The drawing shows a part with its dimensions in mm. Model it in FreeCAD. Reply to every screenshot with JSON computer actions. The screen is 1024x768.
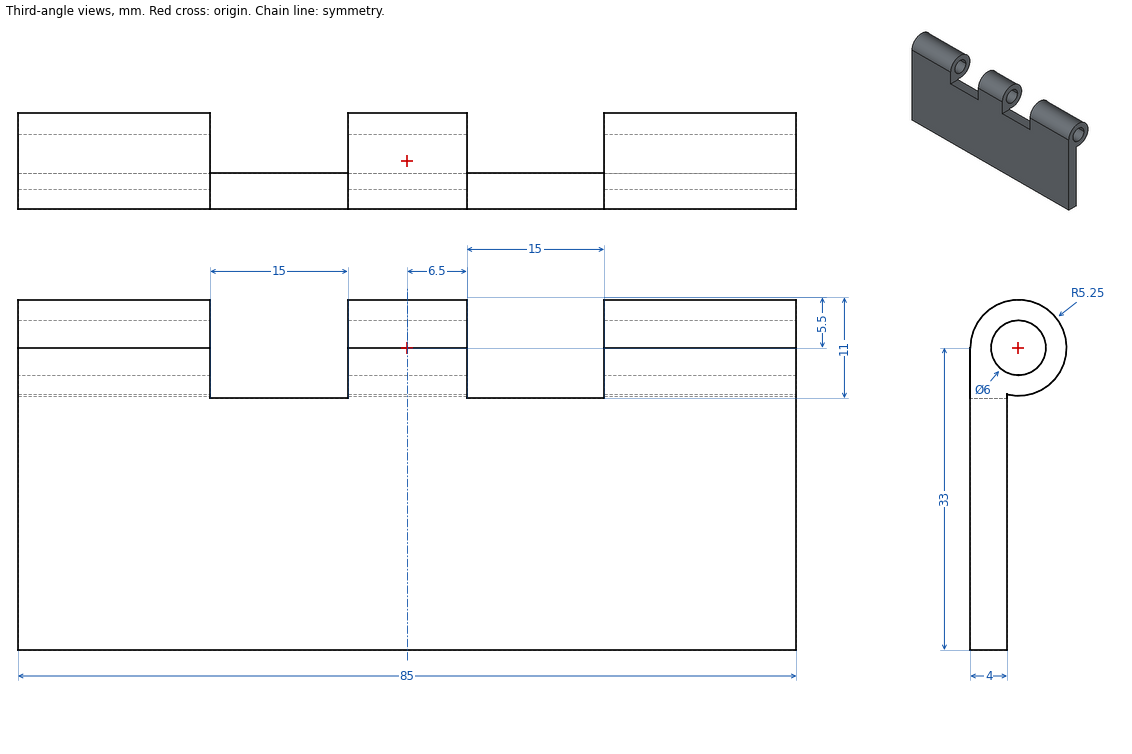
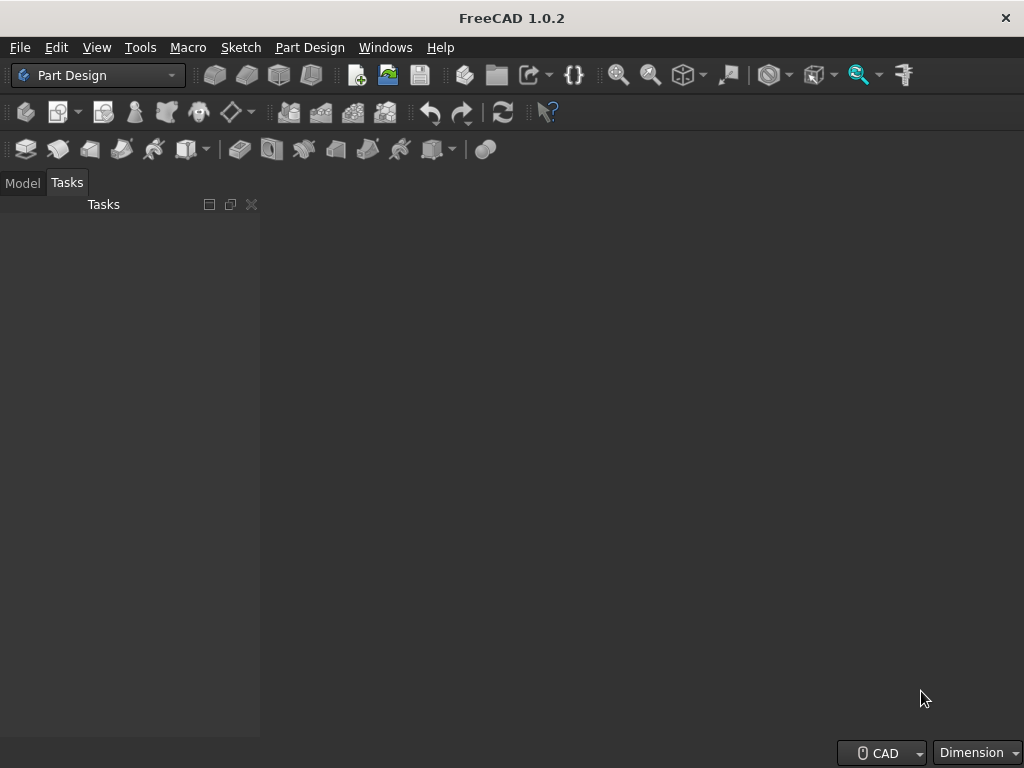
{"action": "left_click", "coordinate": [356, 76]}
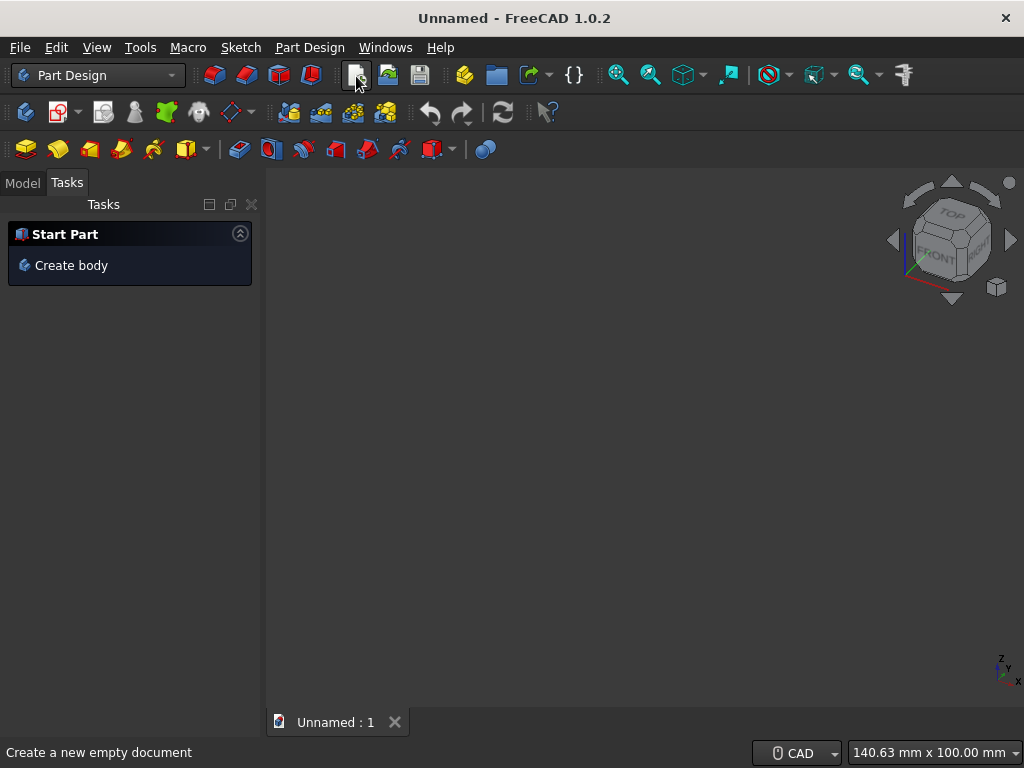
{"action": "left_click", "coordinate": [58, 112]}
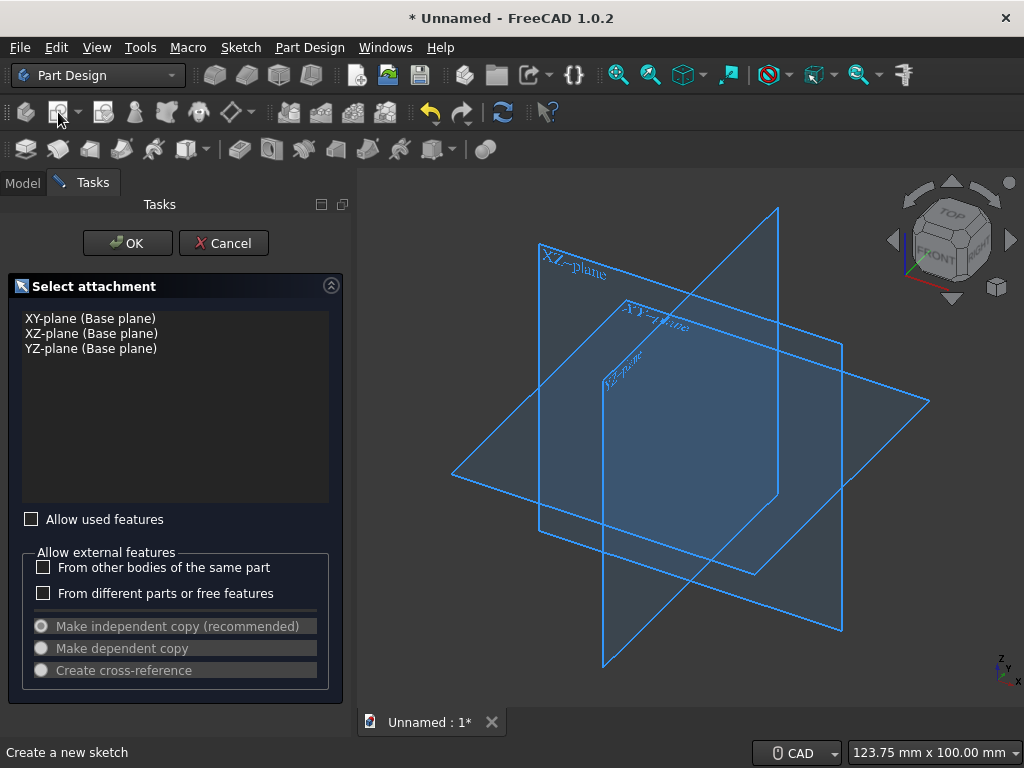
{"action": "left_click", "coordinate": [82, 348]}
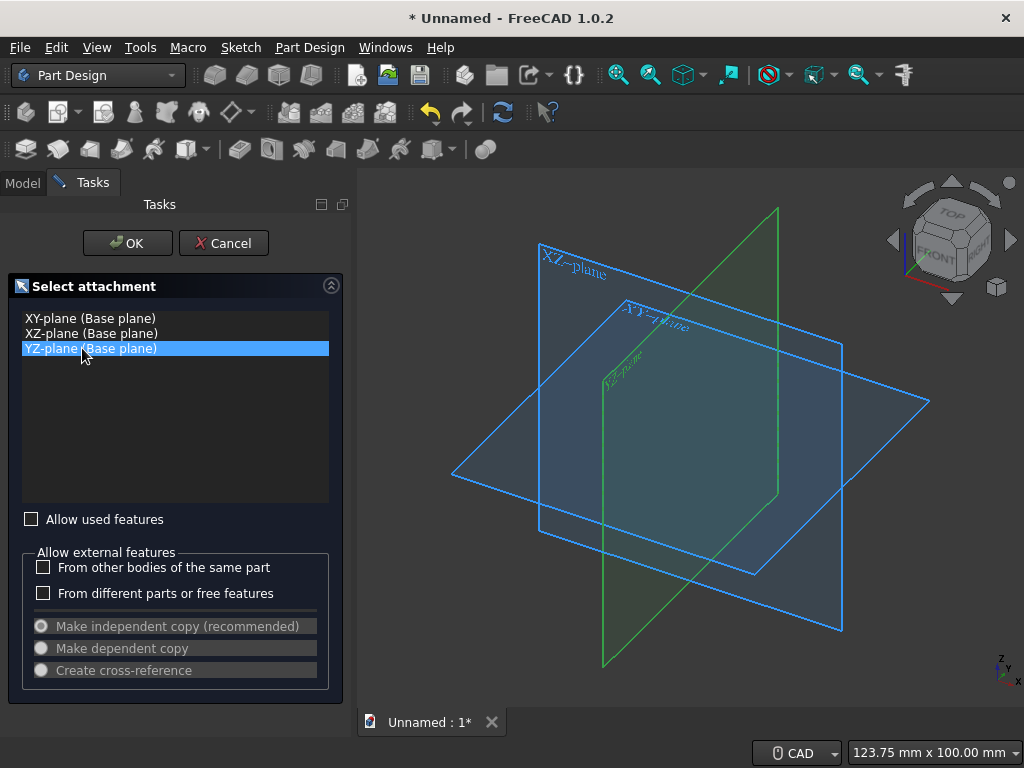
{"action": "left_click", "coordinate": [128, 243]}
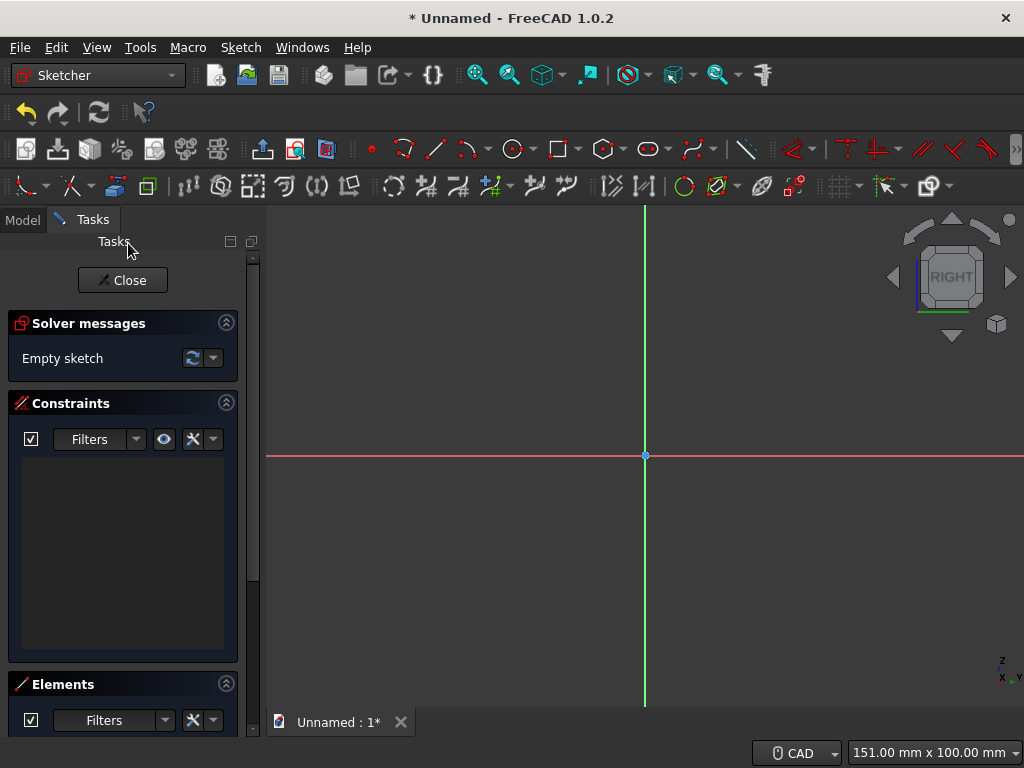
{"action": "scroll", "coordinate": [722, 622], "scroll_direction": "up", "scroll_amount": 3}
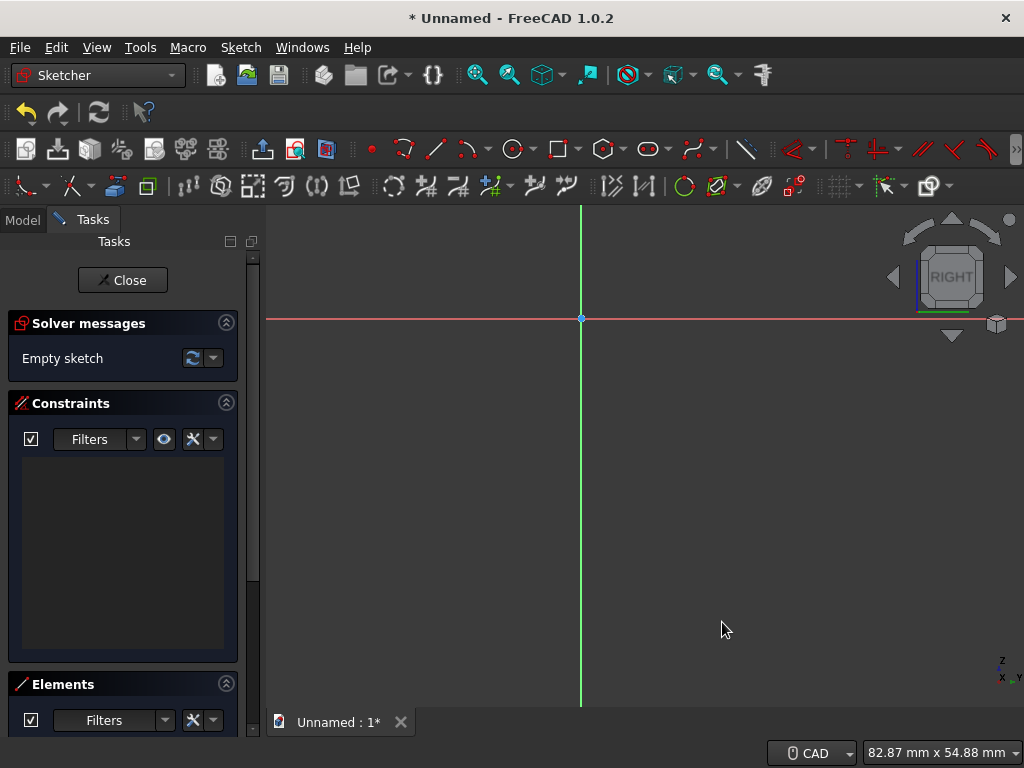
{"action": "left_click", "coordinate": [404, 150]}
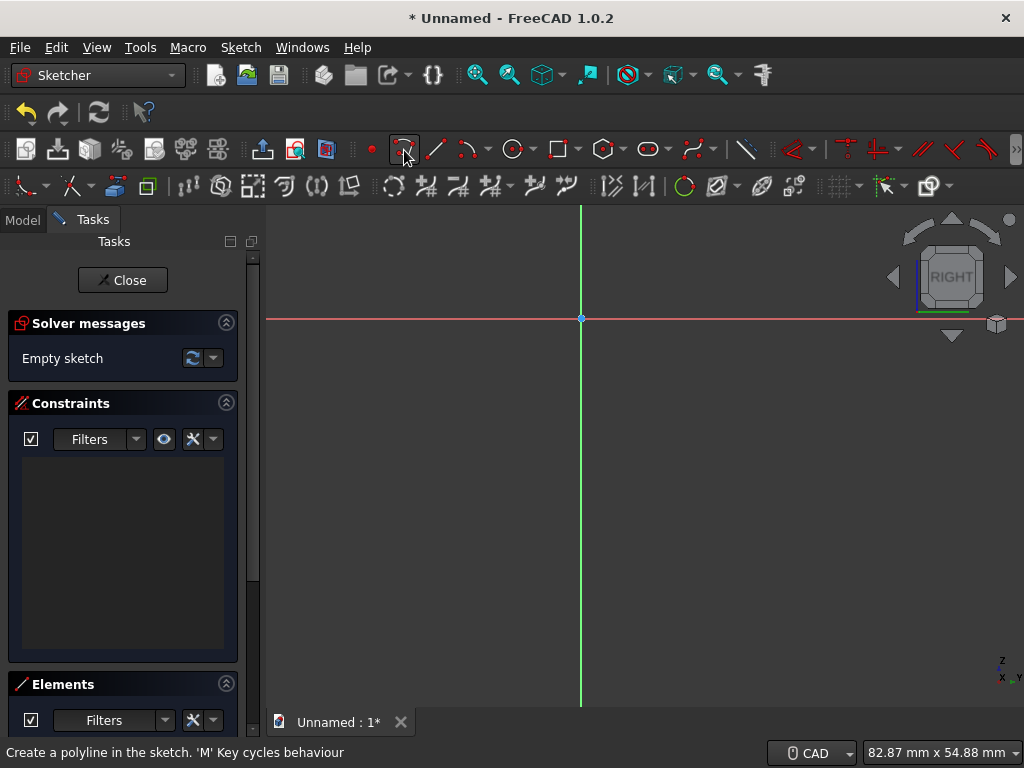
{"action": "left_click", "coordinate": [533, 319]}
{"action": "left_click", "coordinate": [533, 621]}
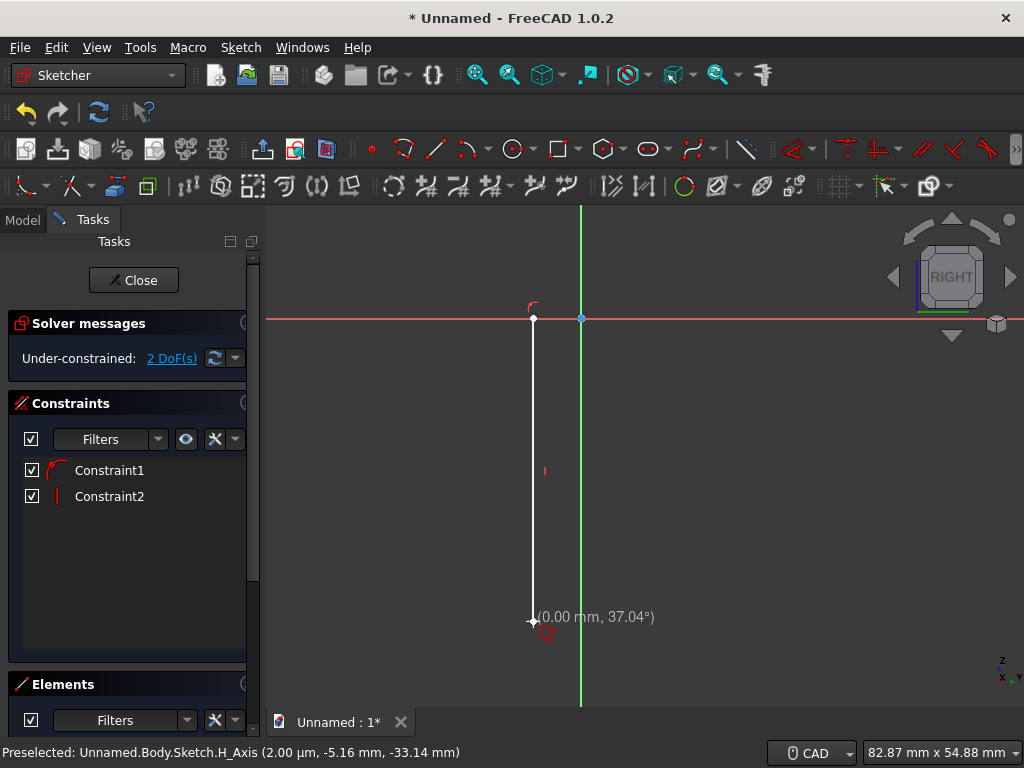
{"action": "scroll", "coordinate": [570, 621], "scroll_direction": "up", "scroll_amount": 2}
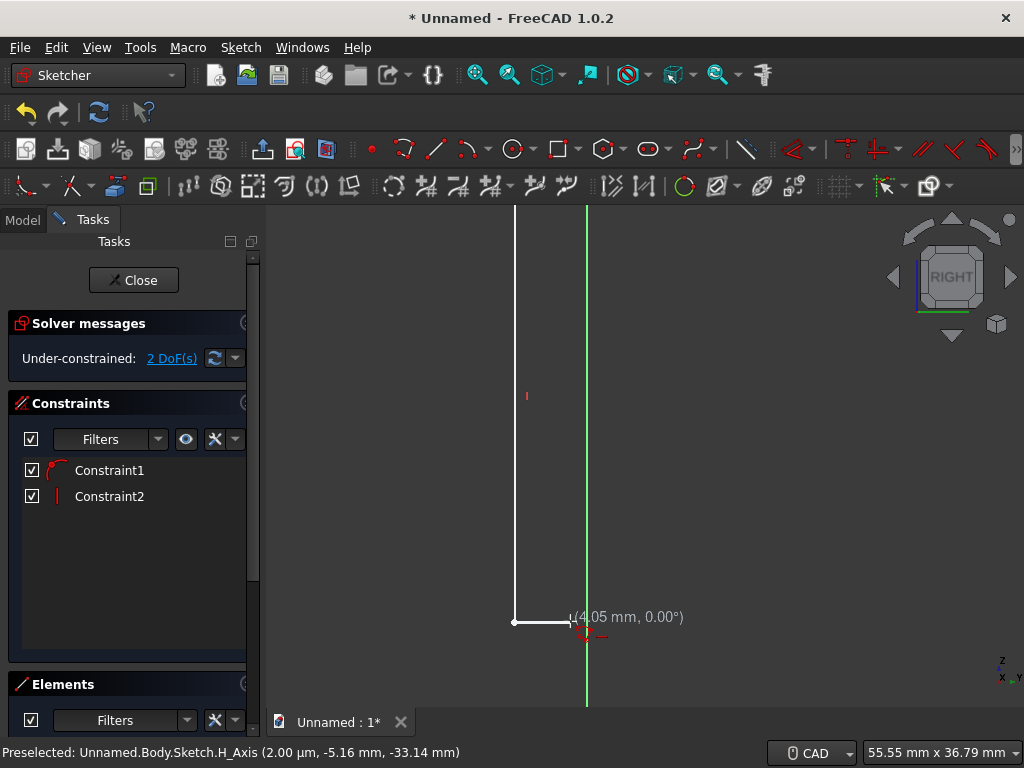
{"action": "left_click", "coordinate": [569, 621]}
{"action": "left_click", "coordinate": [569, 239]}
{"action": "right_click", "coordinate": [569, 239]}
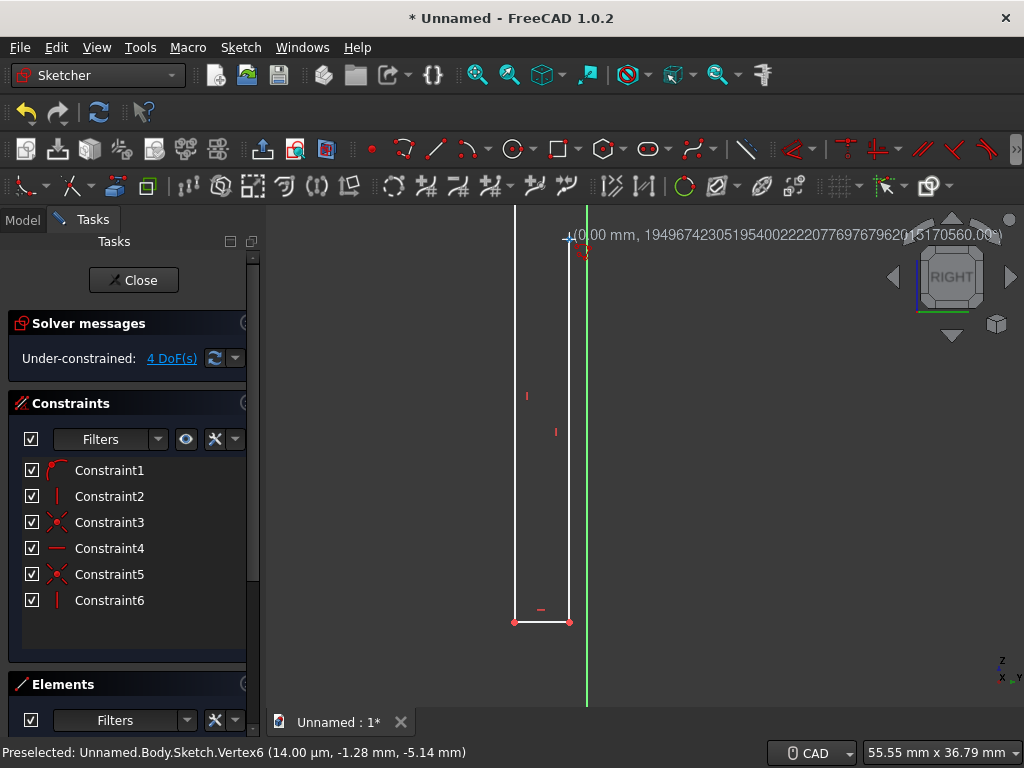
{"action": "key", "text": "g 3 a"}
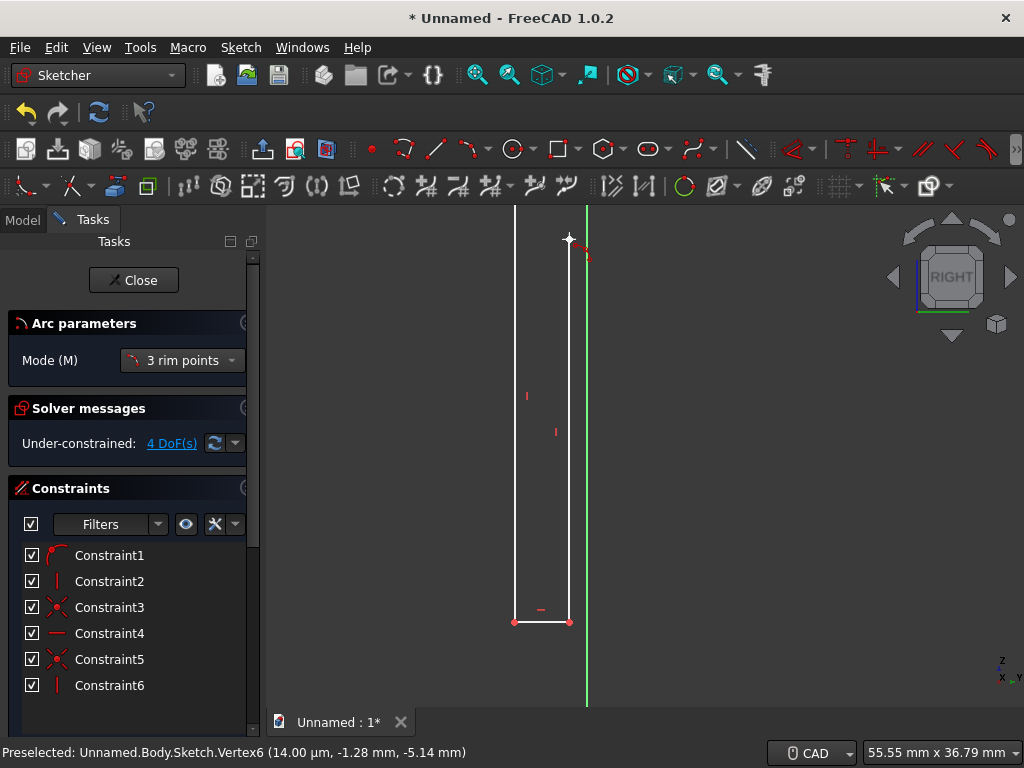
{"action": "left_click", "coordinate": [569, 240]}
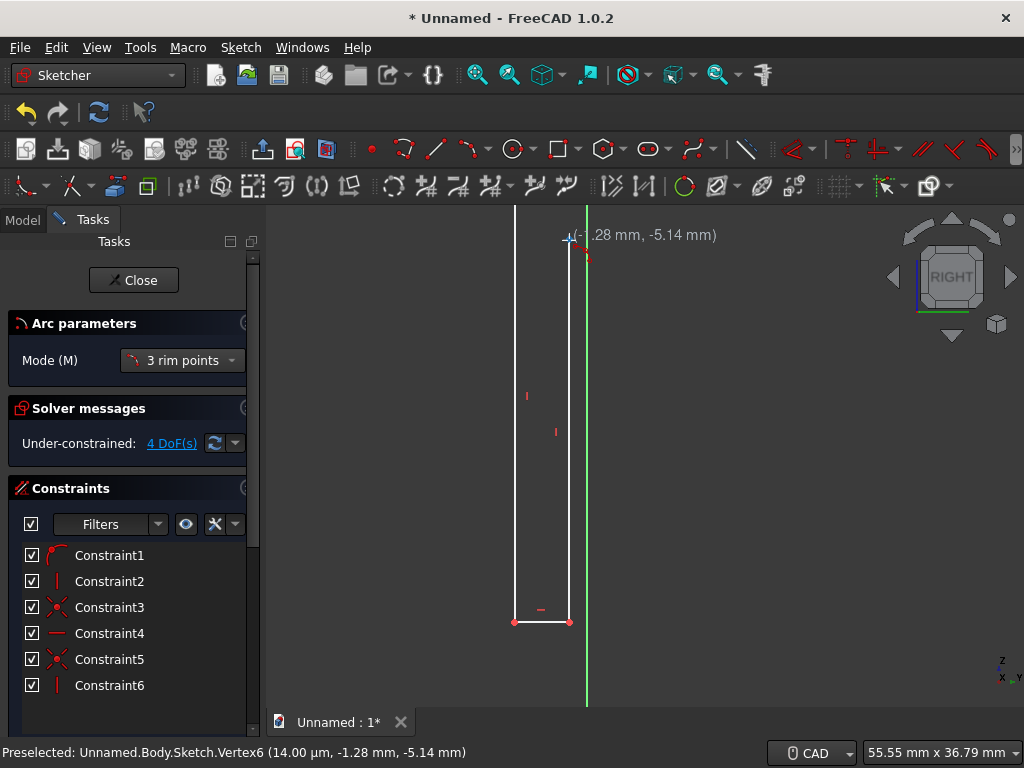
{"action": "scroll", "coordinate": [572, 625], "scroll_direction": "down", "scroll_amount": 2}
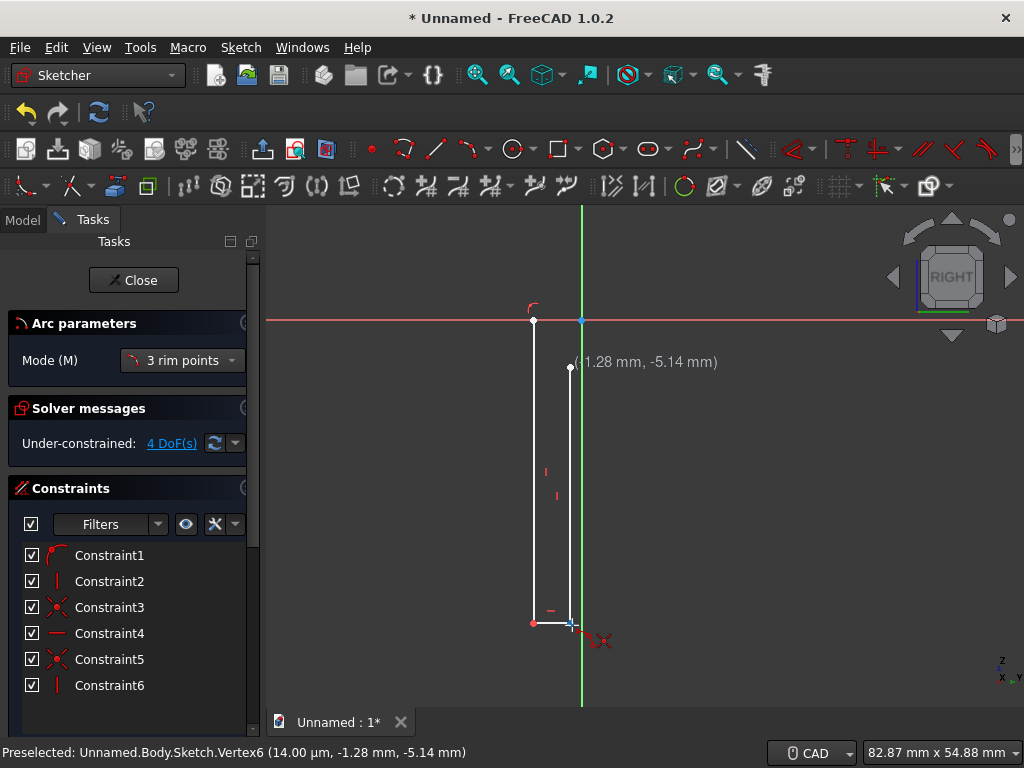
{"action": "left_click", "coordinate": [534, 320]}
{"action": "left_click", "coordinate": [620, 291]}
{"action": "key", "text": "Escape"}